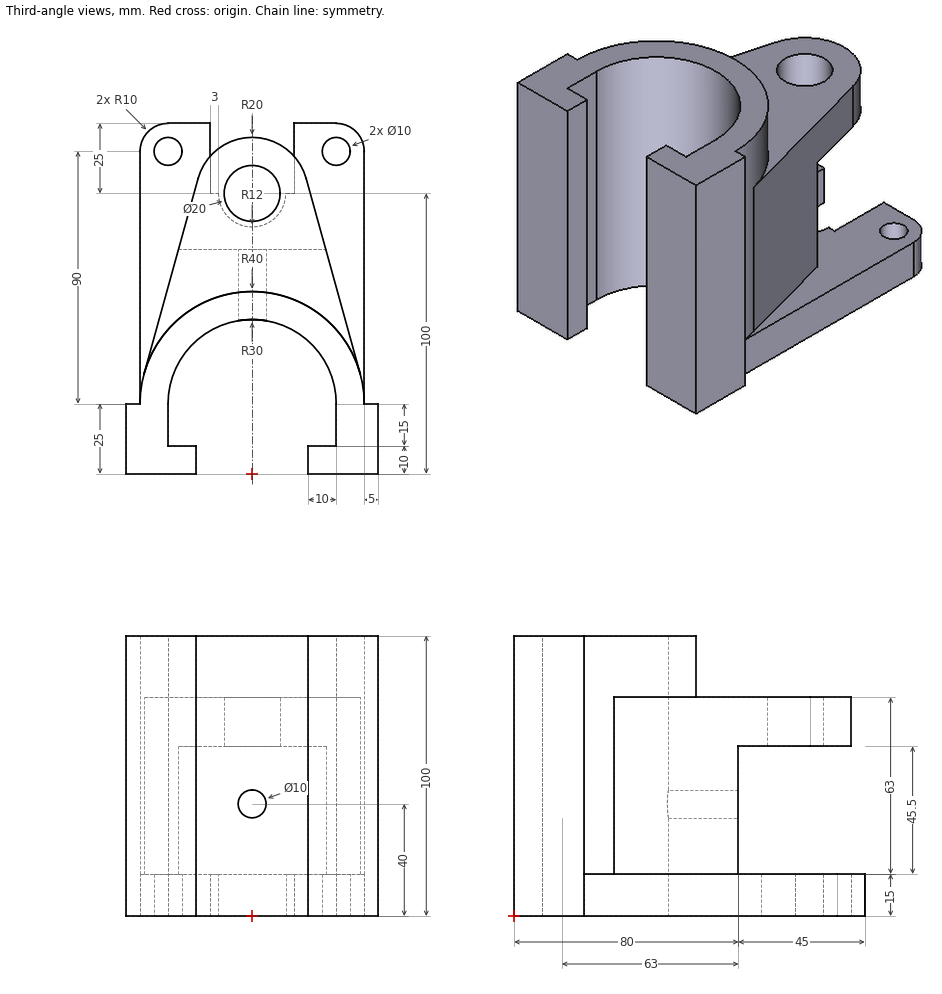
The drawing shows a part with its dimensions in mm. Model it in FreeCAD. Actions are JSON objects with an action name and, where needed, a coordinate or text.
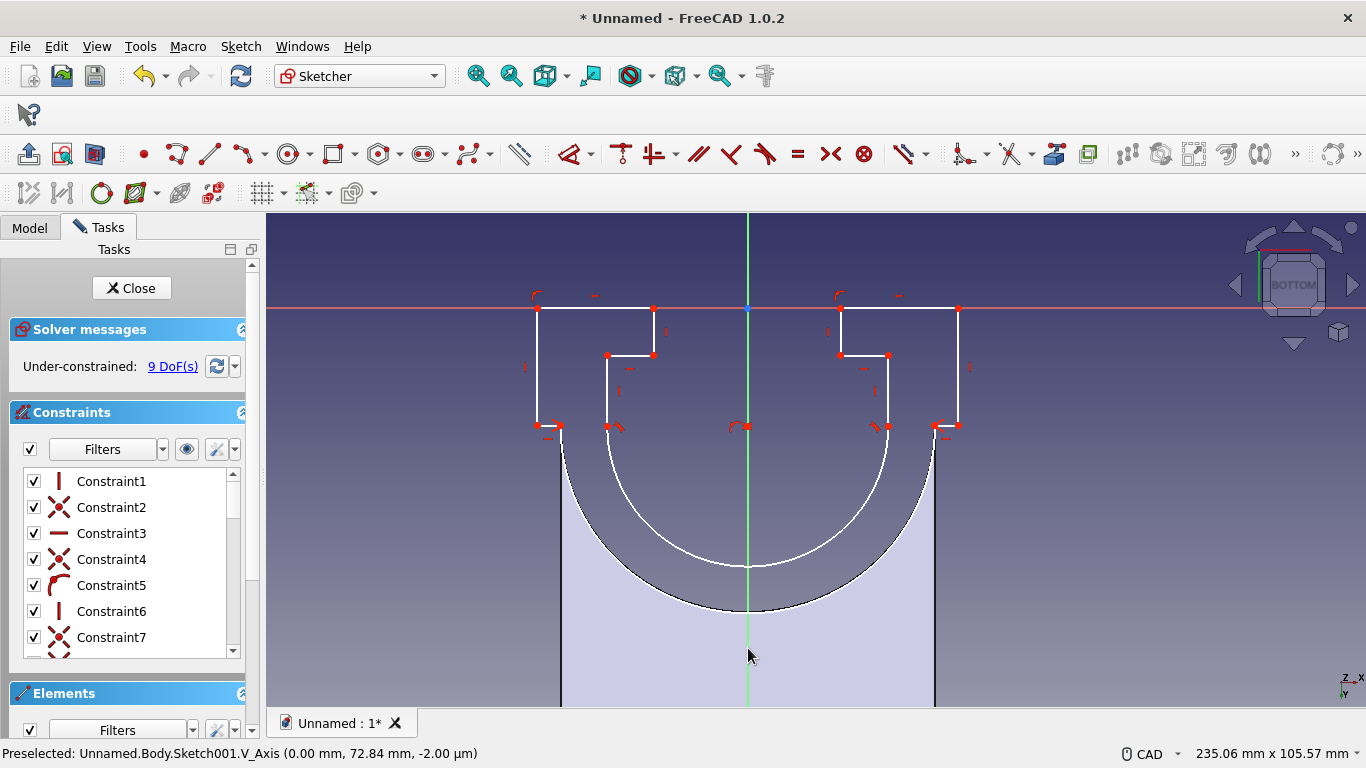
{"action": "left_click", "coordinate": [841, 356]}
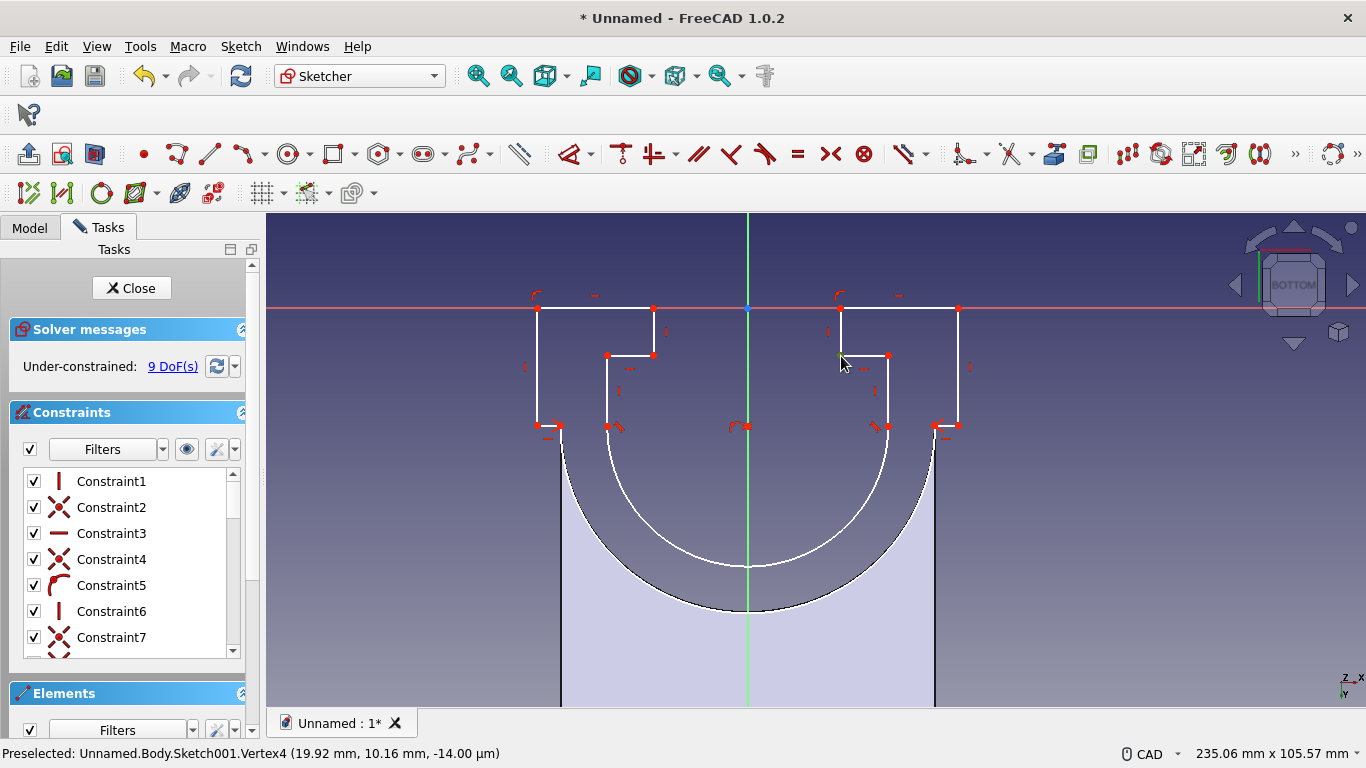
{"action": "left_click", "coordinate": [654, 356]}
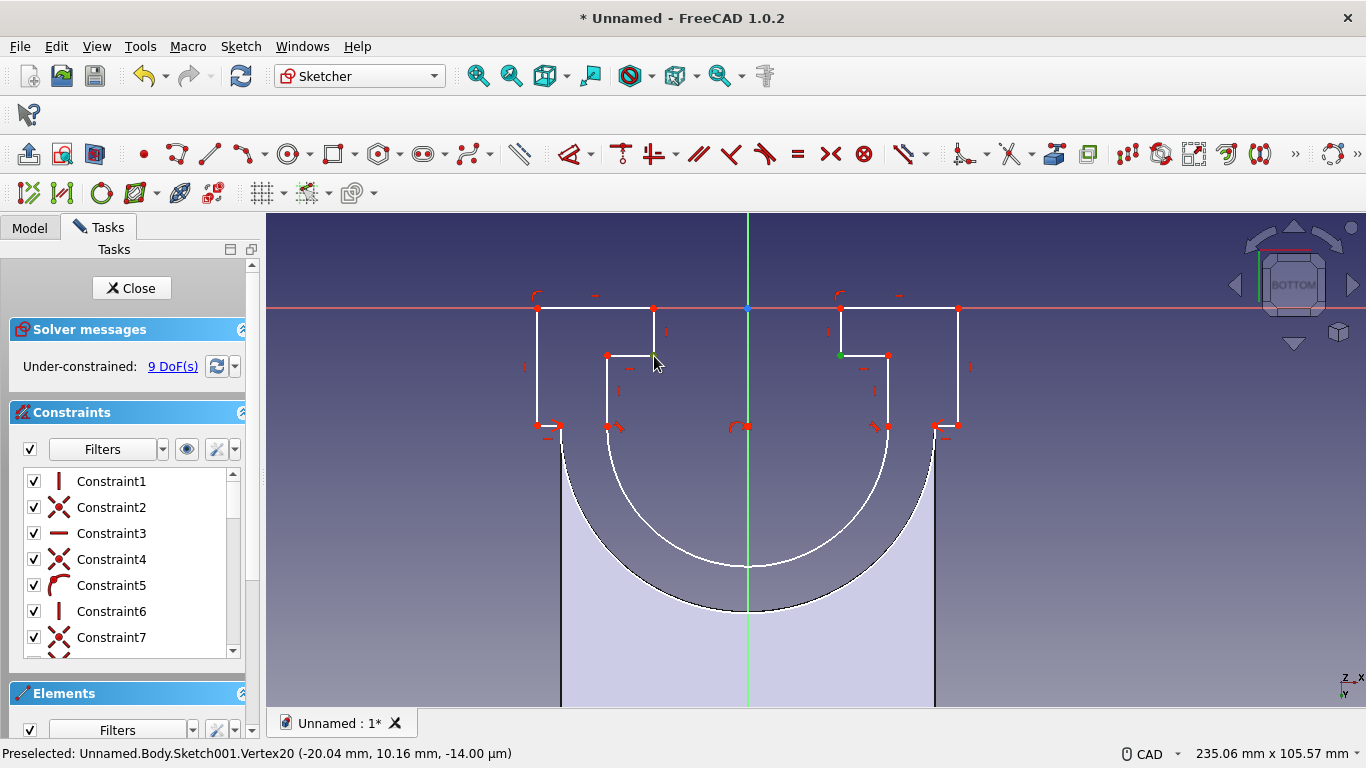
{"action": "left_click", "coordinate": [748, 648]}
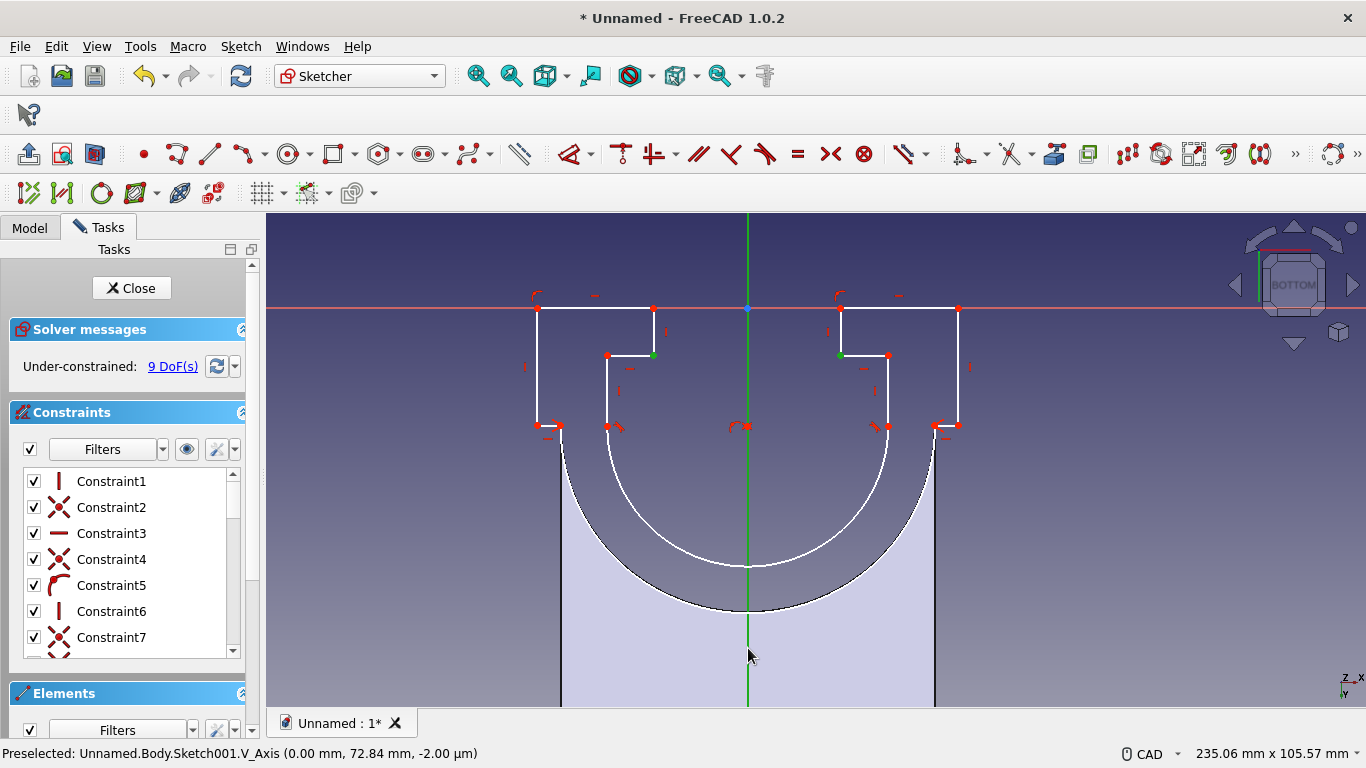
{"action": "key", "text": "s"}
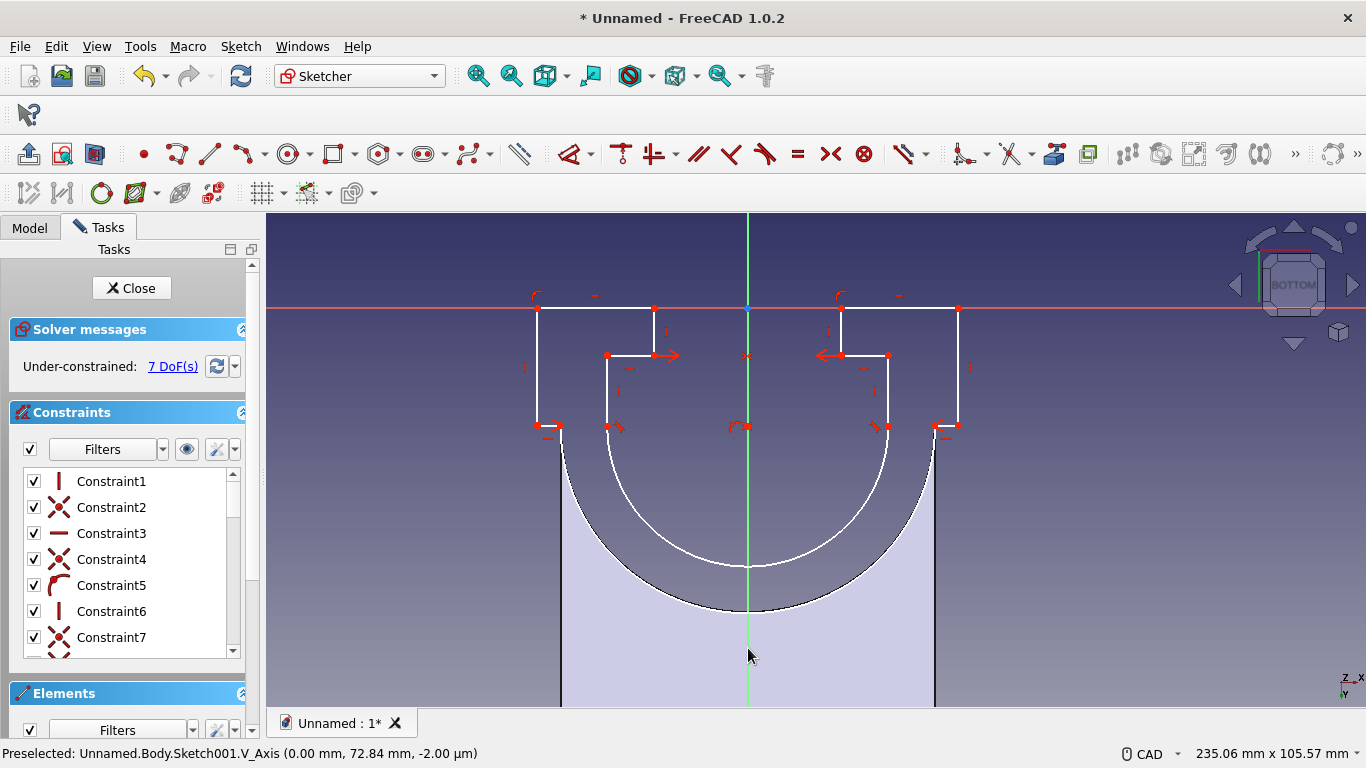
{"action": "key", "text": "d"}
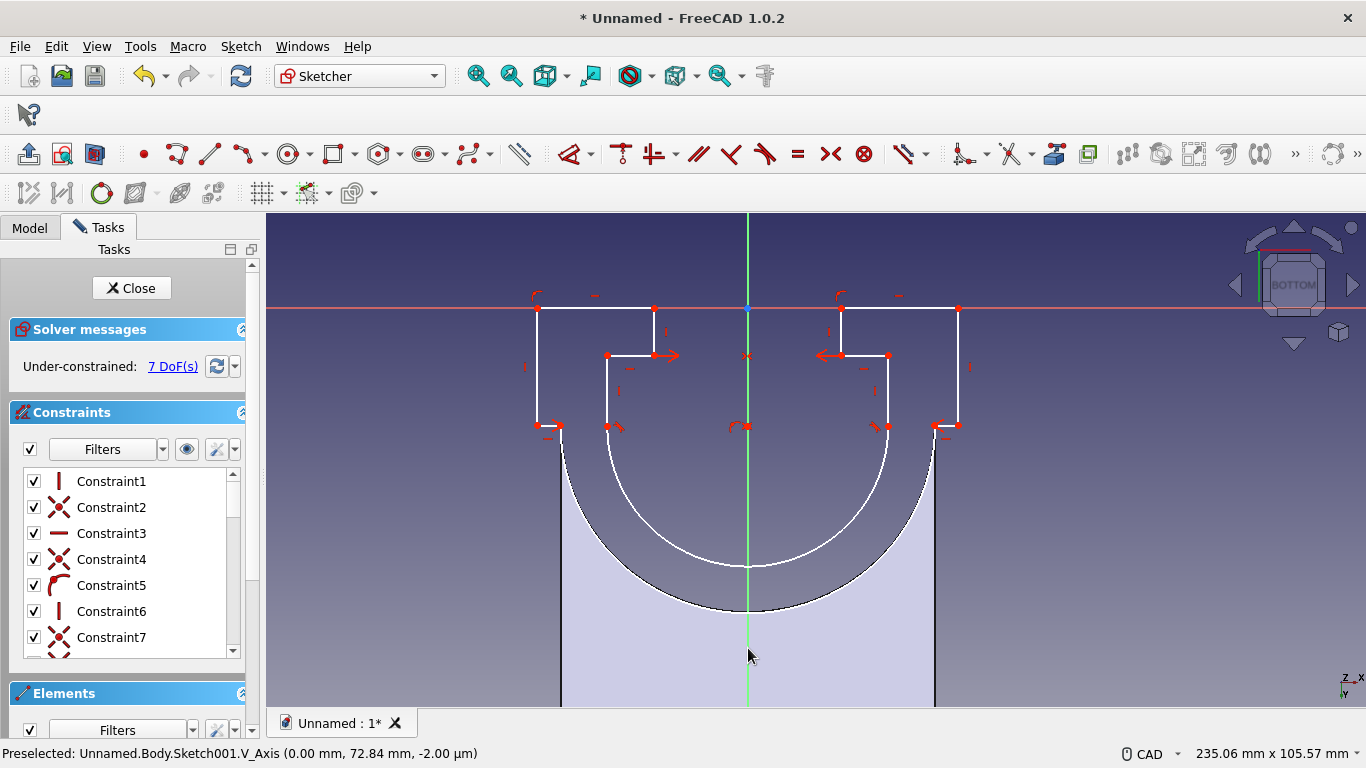
{"action": "left_click", "coordinate": [638, 577]}
{"action": "left_click", "coordinate": [619, 603]}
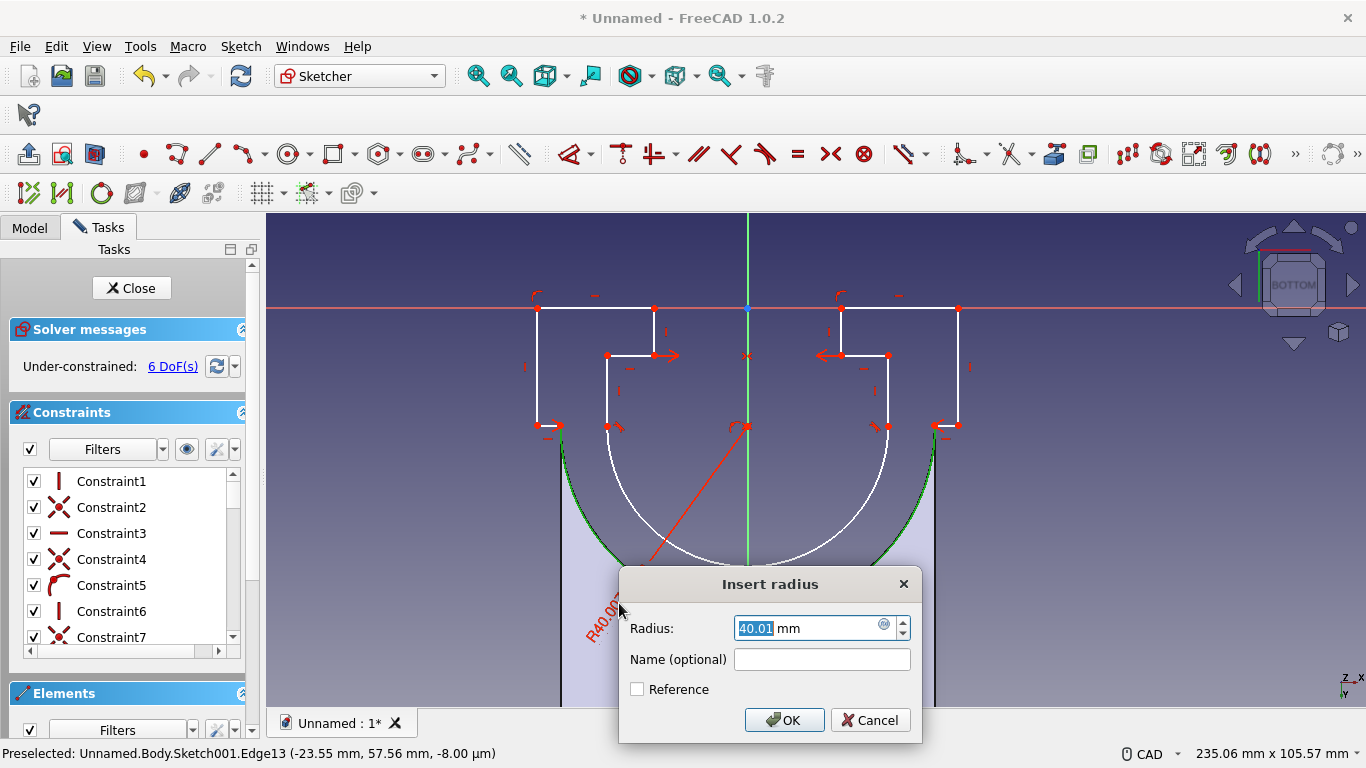
{"action": "type", "text": "40"}
{"action": "key", "text": "Return"}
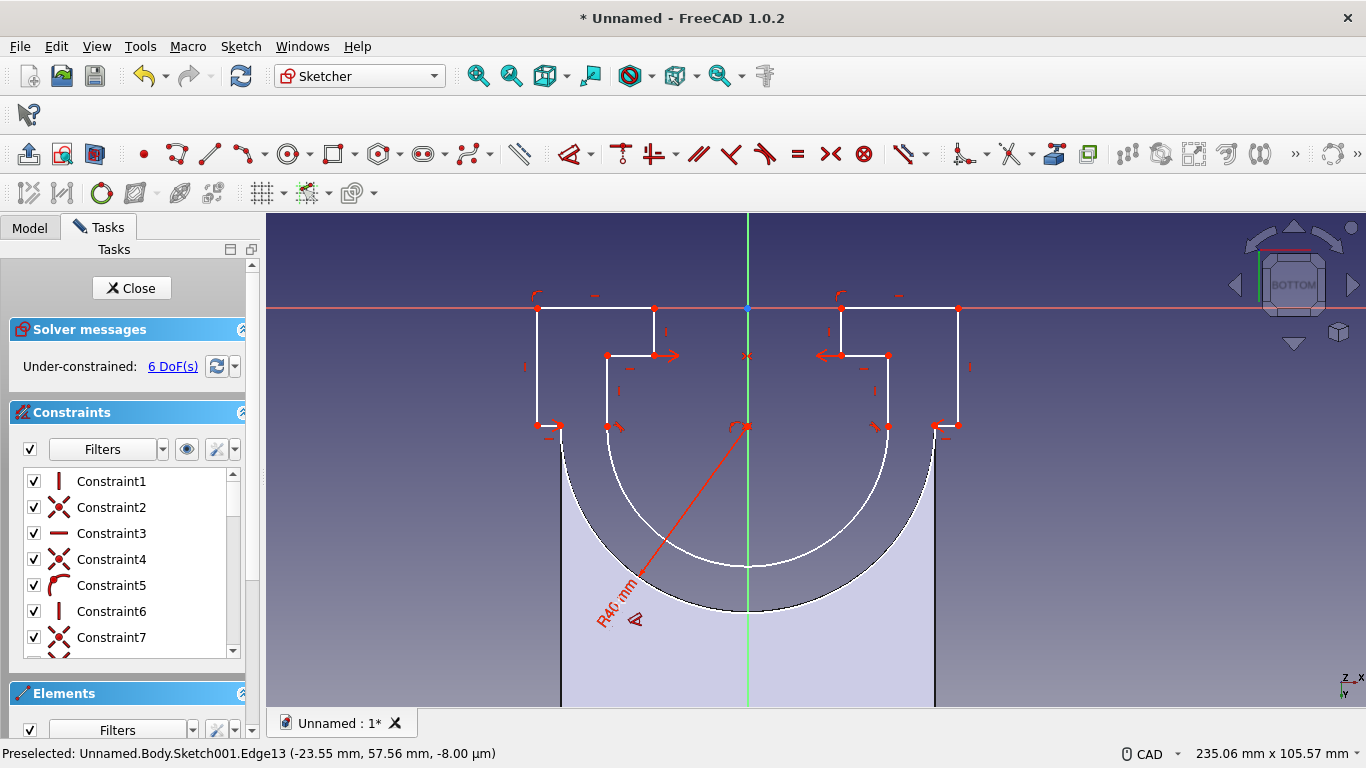
{"action": "left_click", "coordinate": [665, 540]}
{"action": "left_click", "coordinate": [646, 566]}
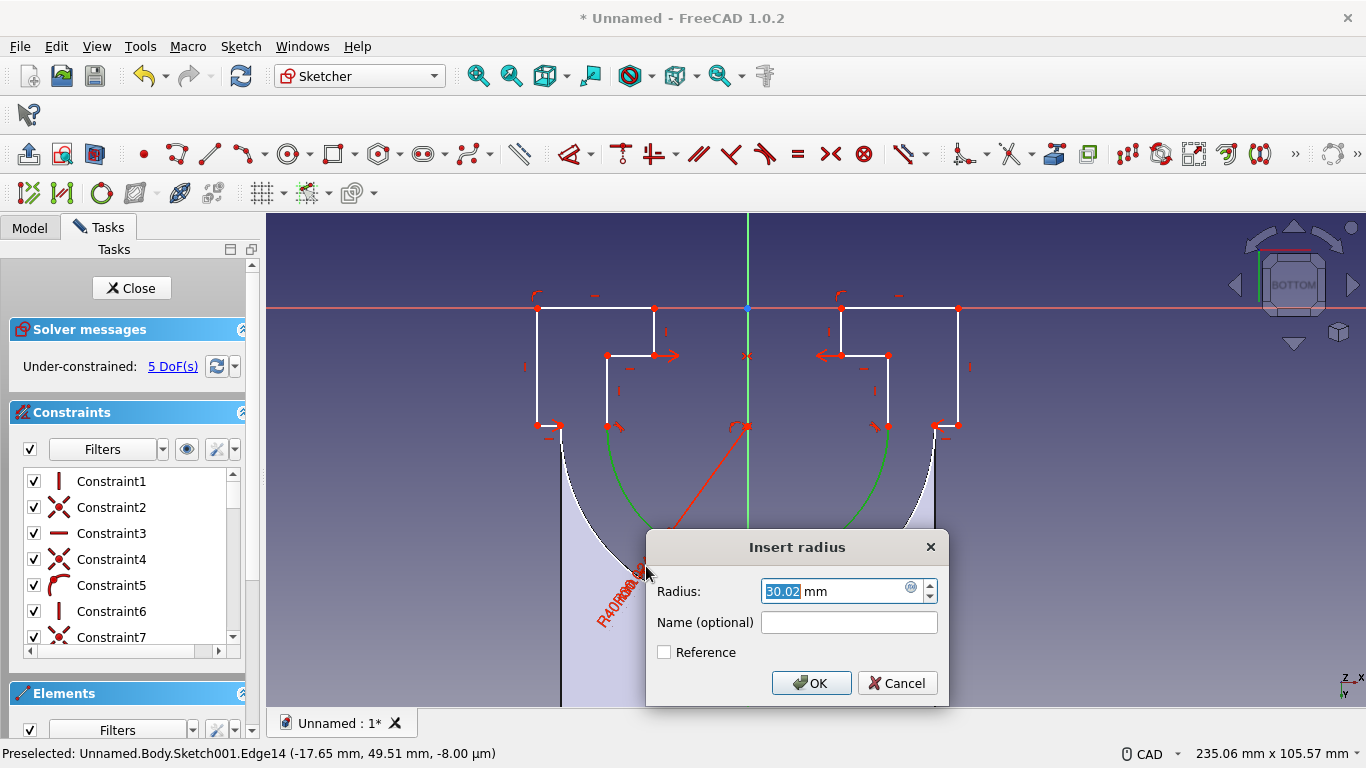
{"action": "type", "text": "30"}
{"action": "key", "text": "Return"}